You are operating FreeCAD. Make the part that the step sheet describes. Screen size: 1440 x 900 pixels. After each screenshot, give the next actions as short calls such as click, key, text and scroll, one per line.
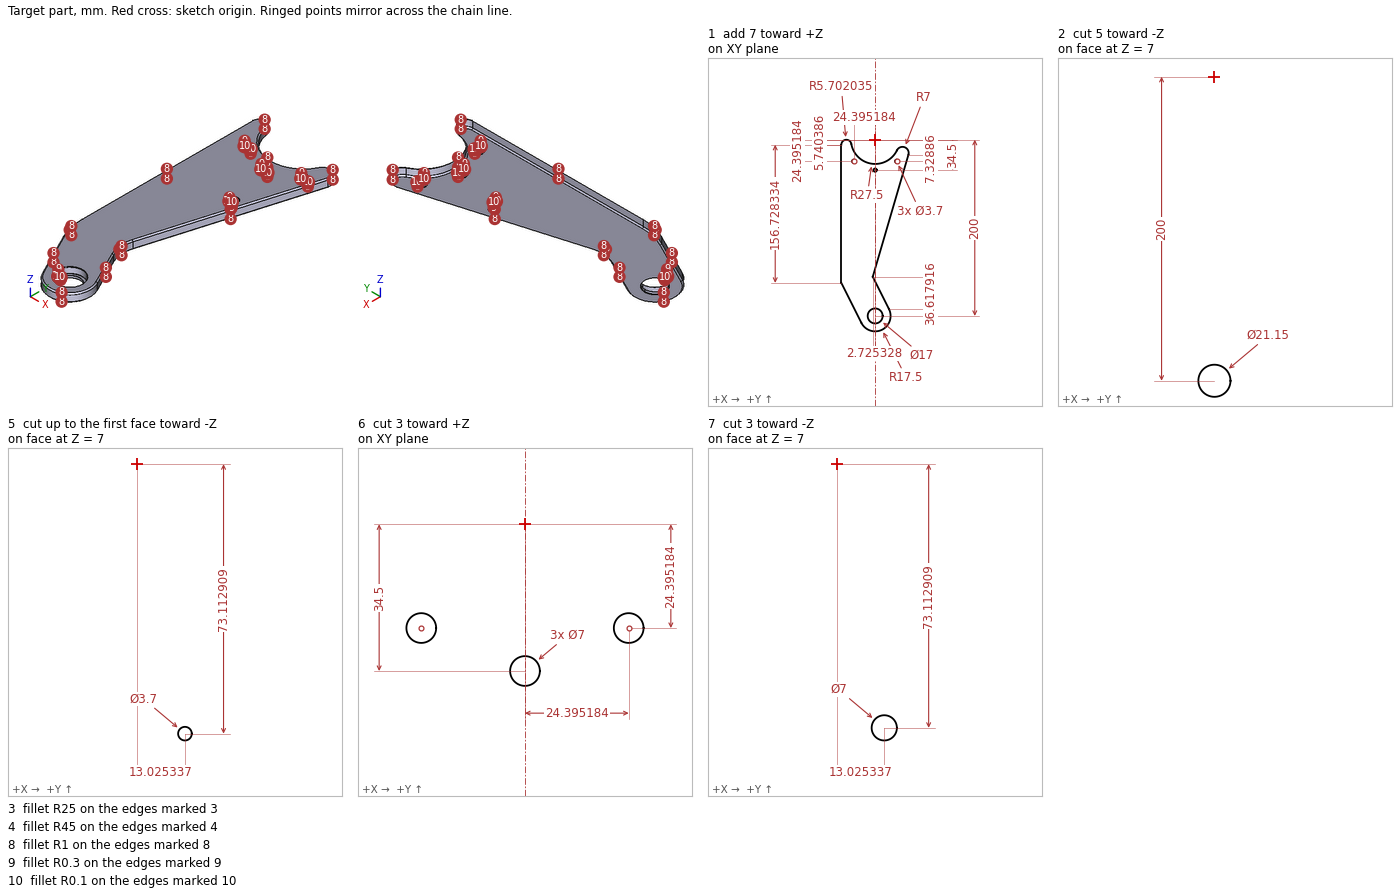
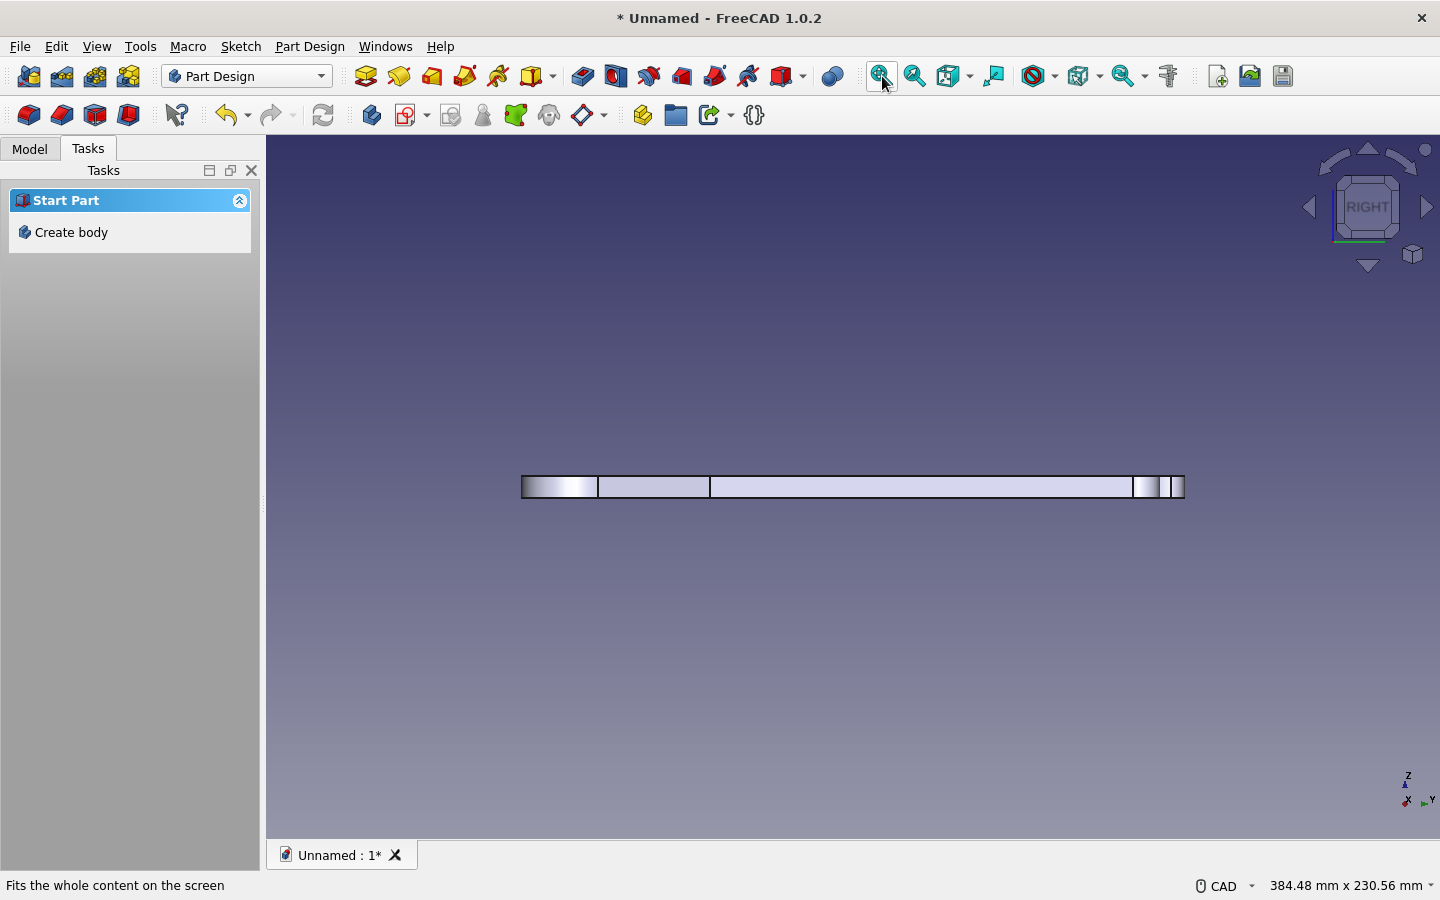
scroll(710, 486, up, 4)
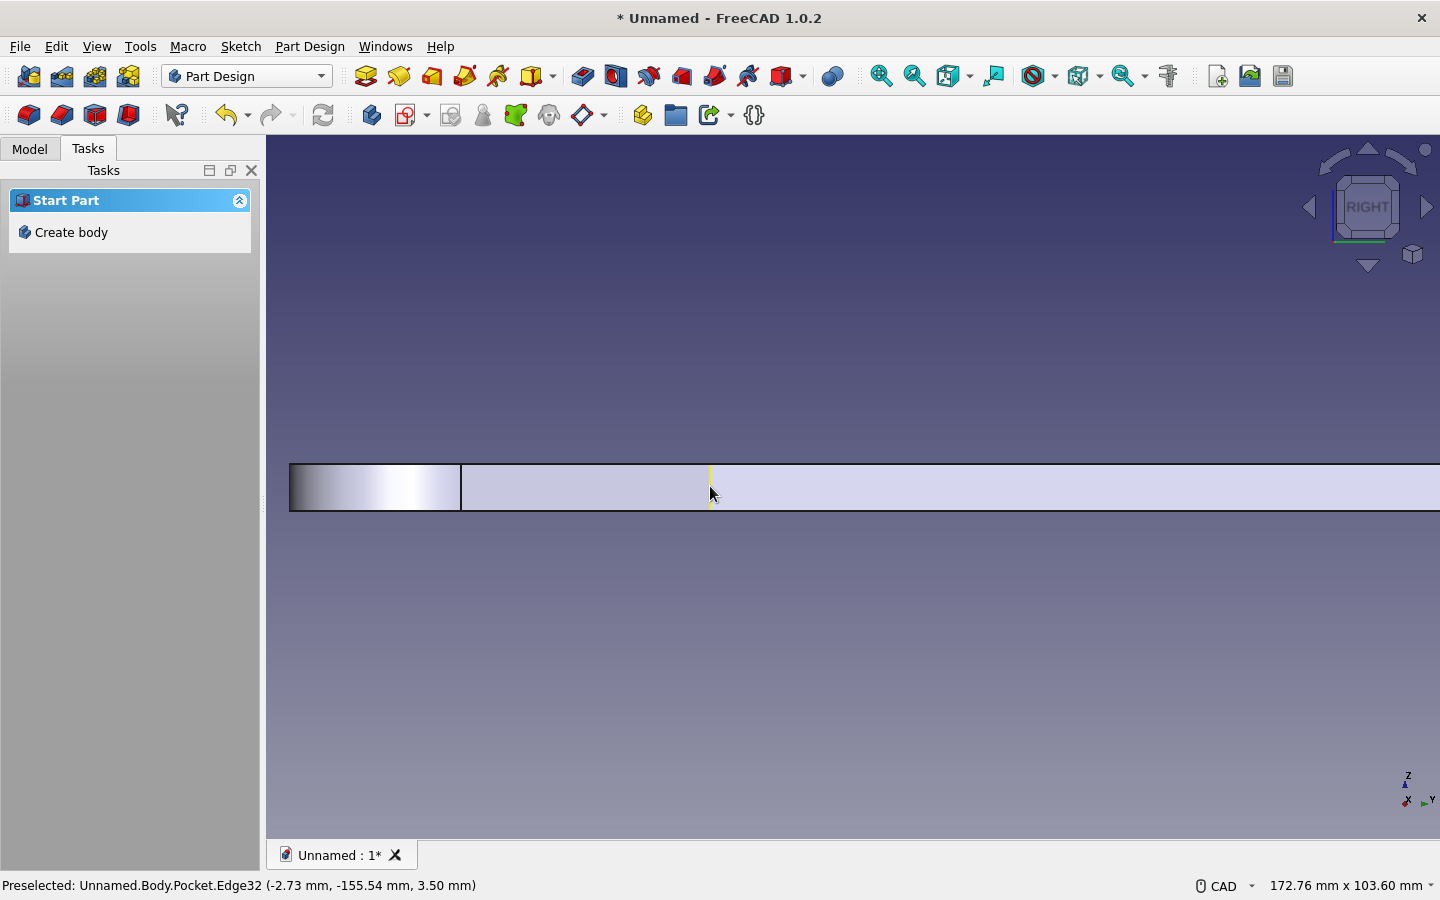
click(882, 76)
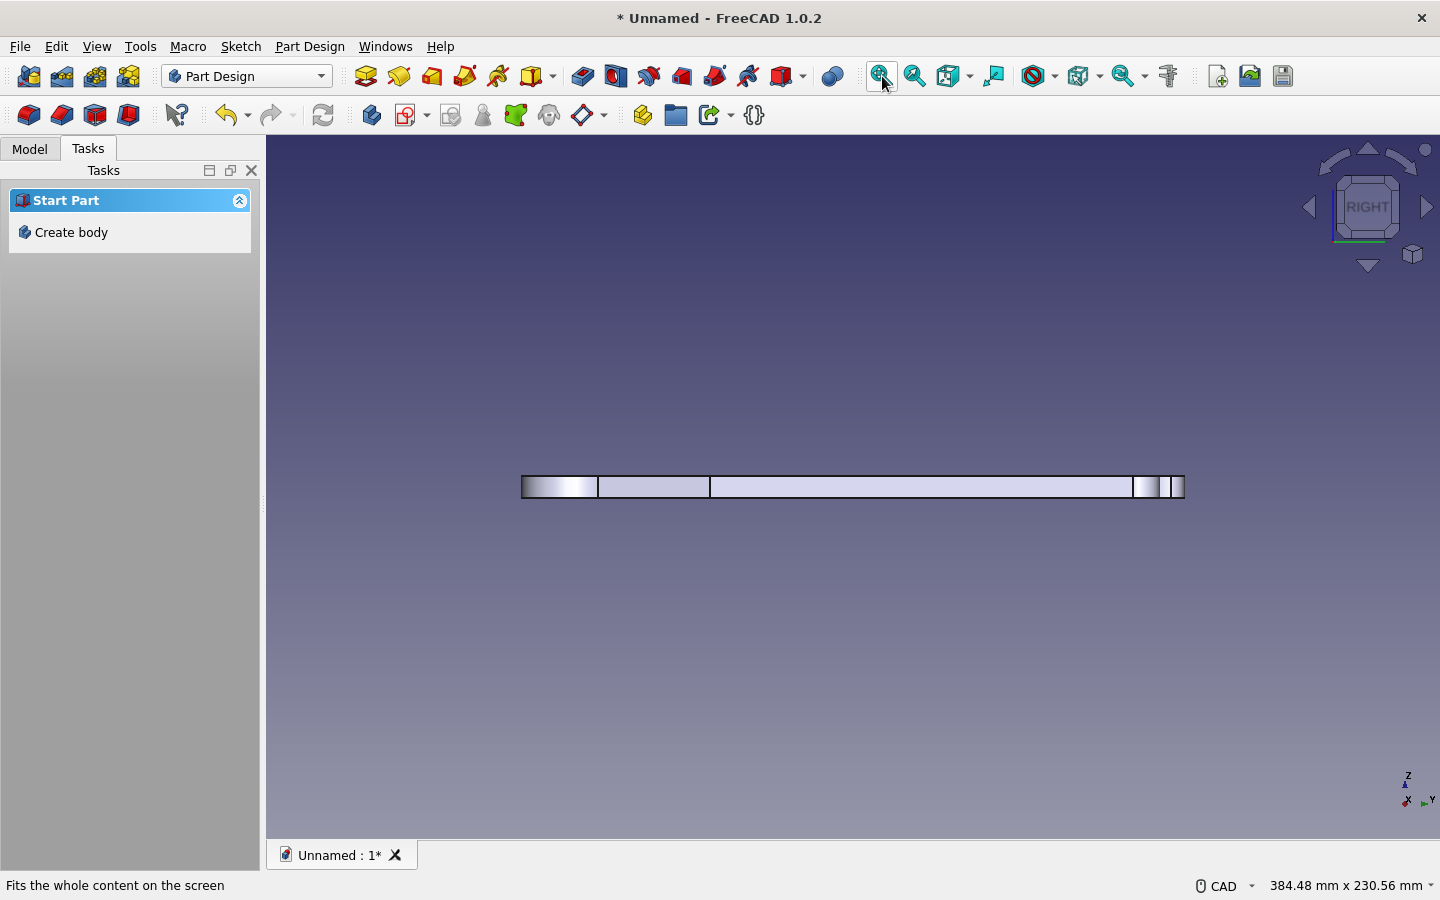
key(5)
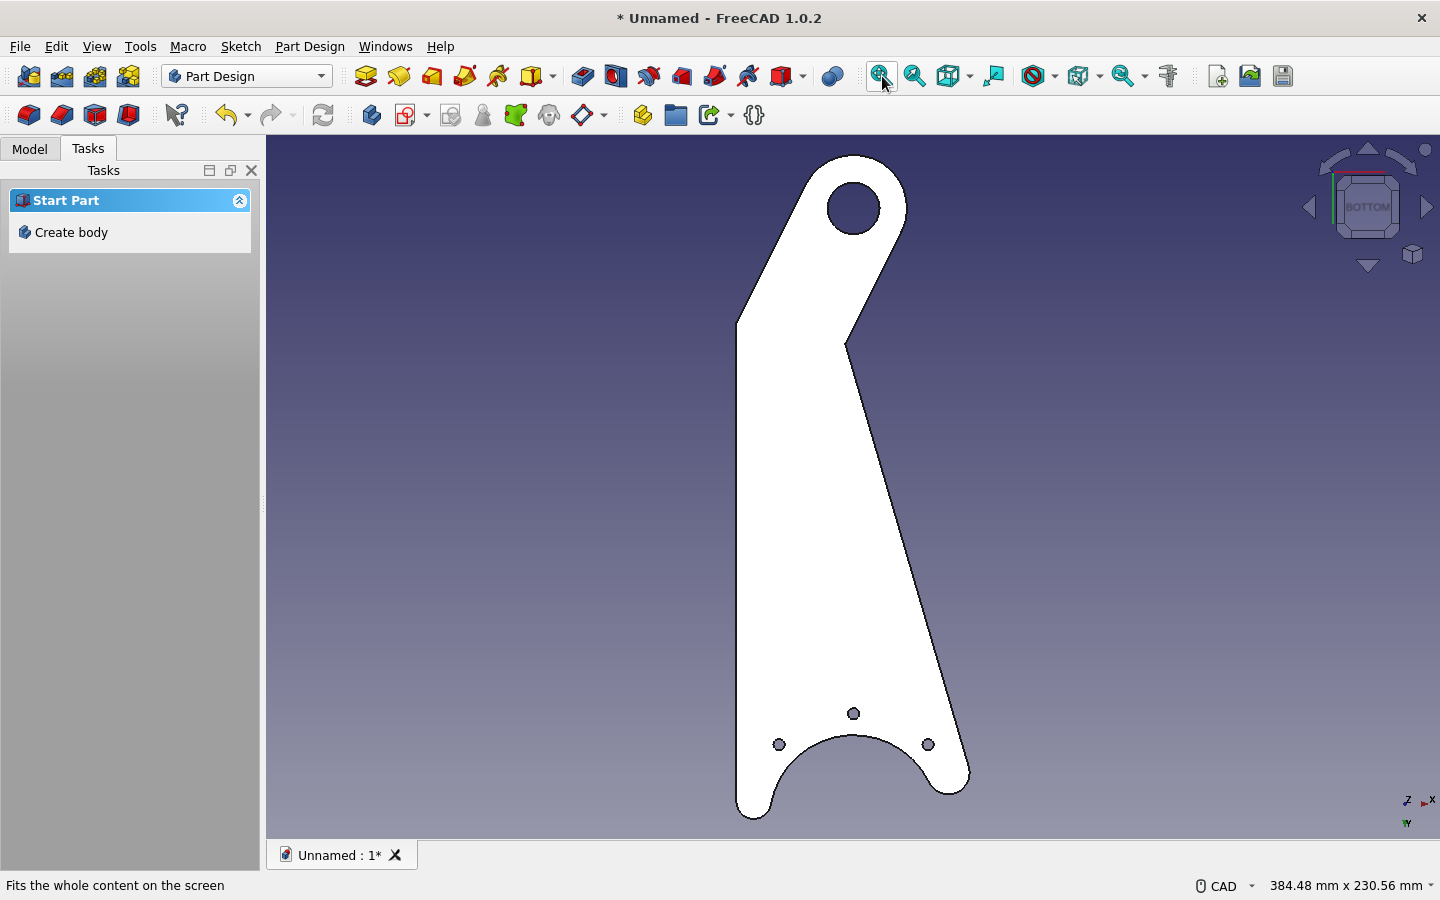
scroll(845, 343, up, 4)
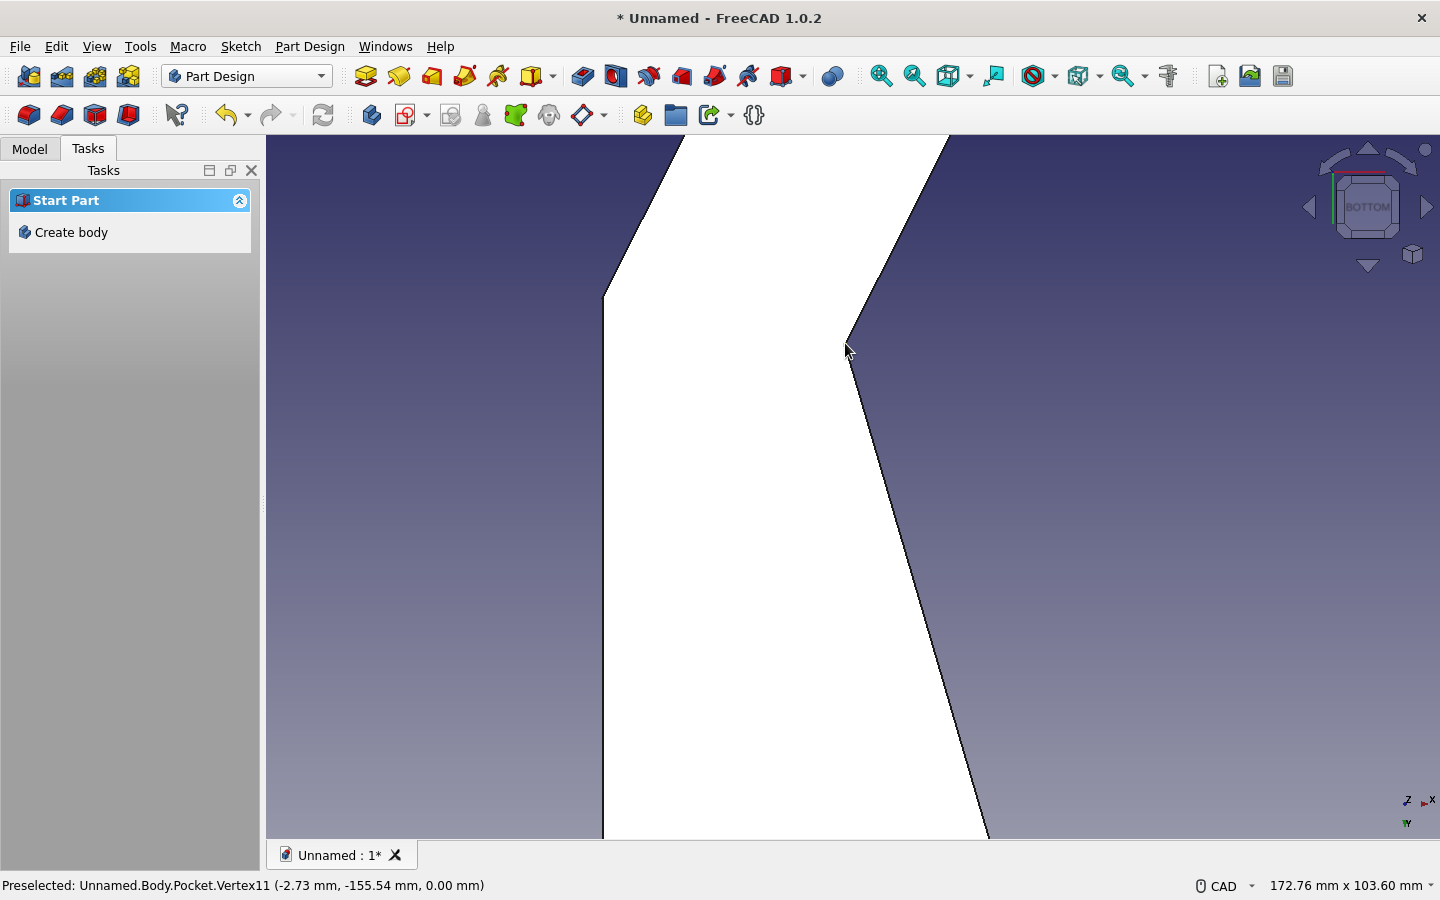
click(882, 76)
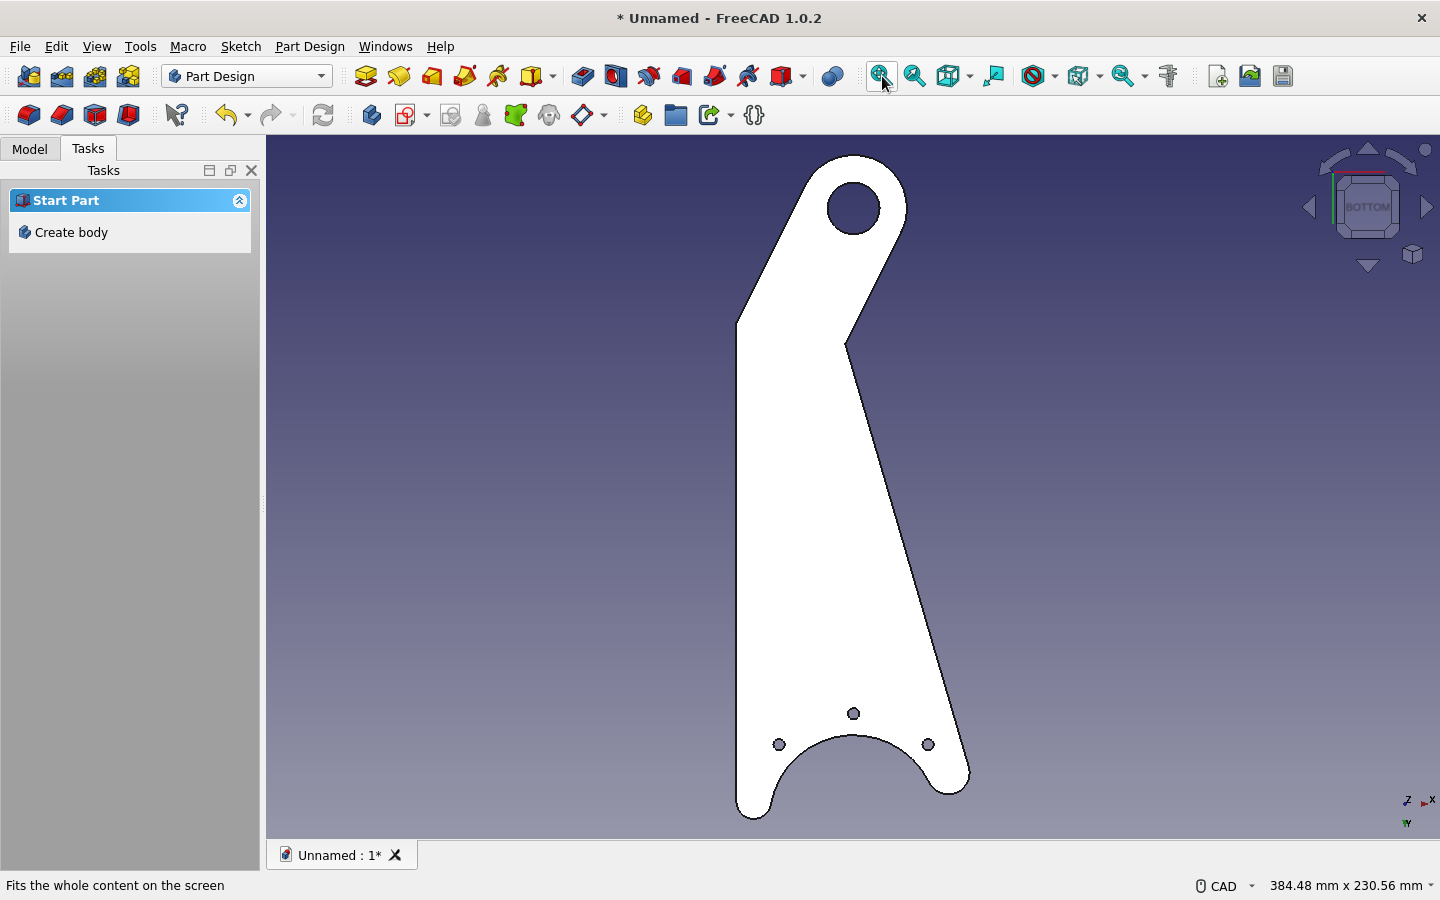
key(4)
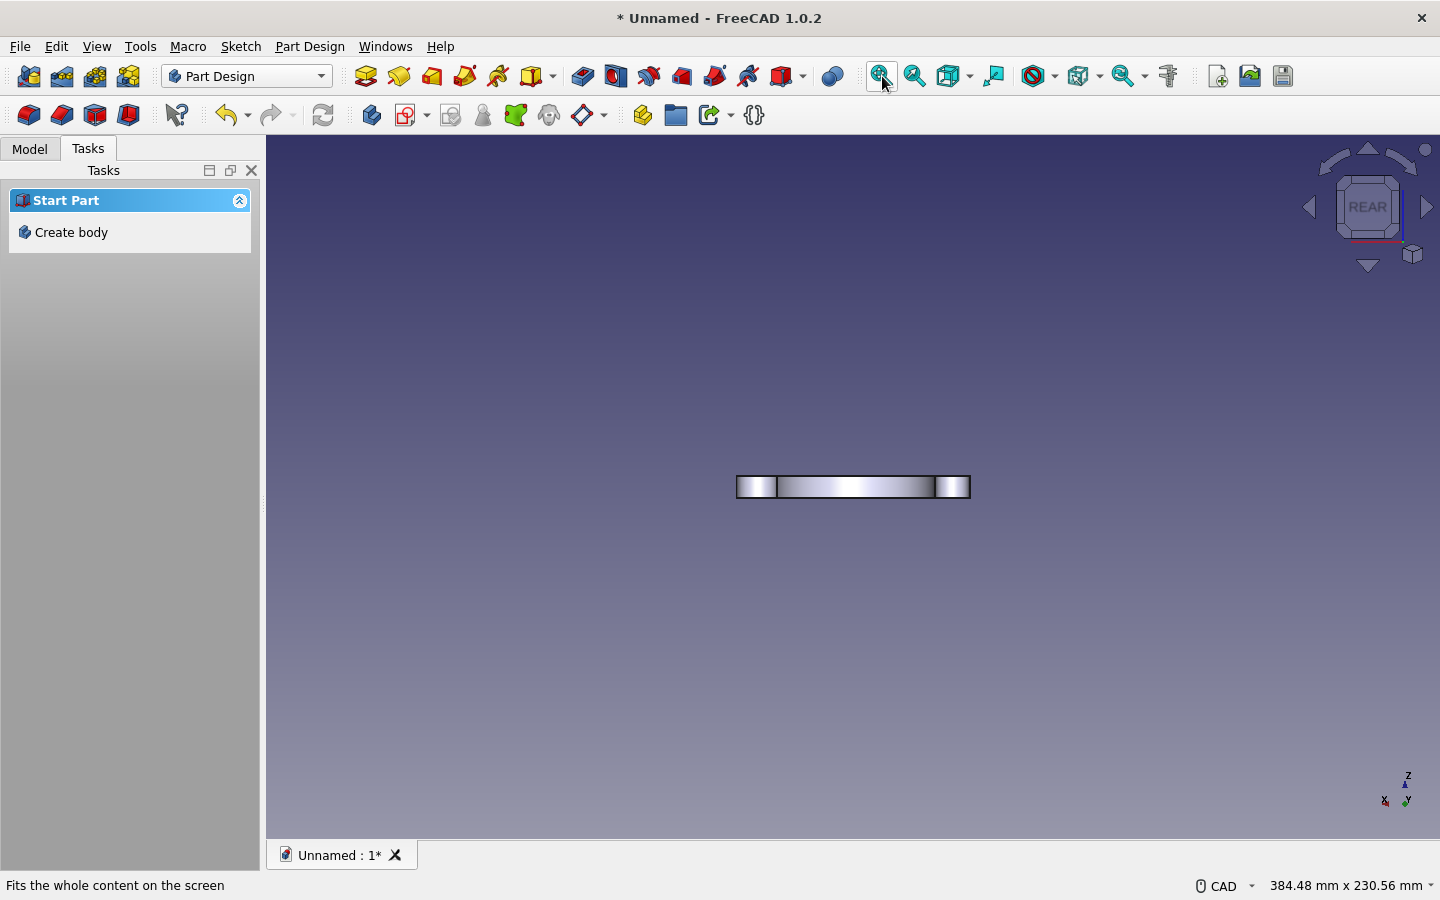
key(v)
key(f)